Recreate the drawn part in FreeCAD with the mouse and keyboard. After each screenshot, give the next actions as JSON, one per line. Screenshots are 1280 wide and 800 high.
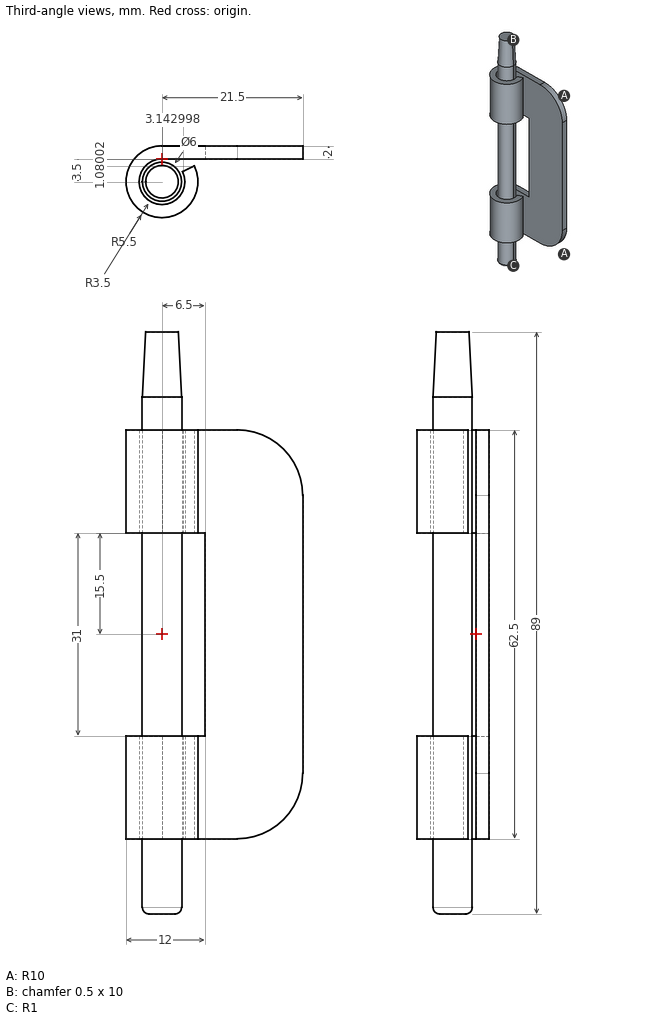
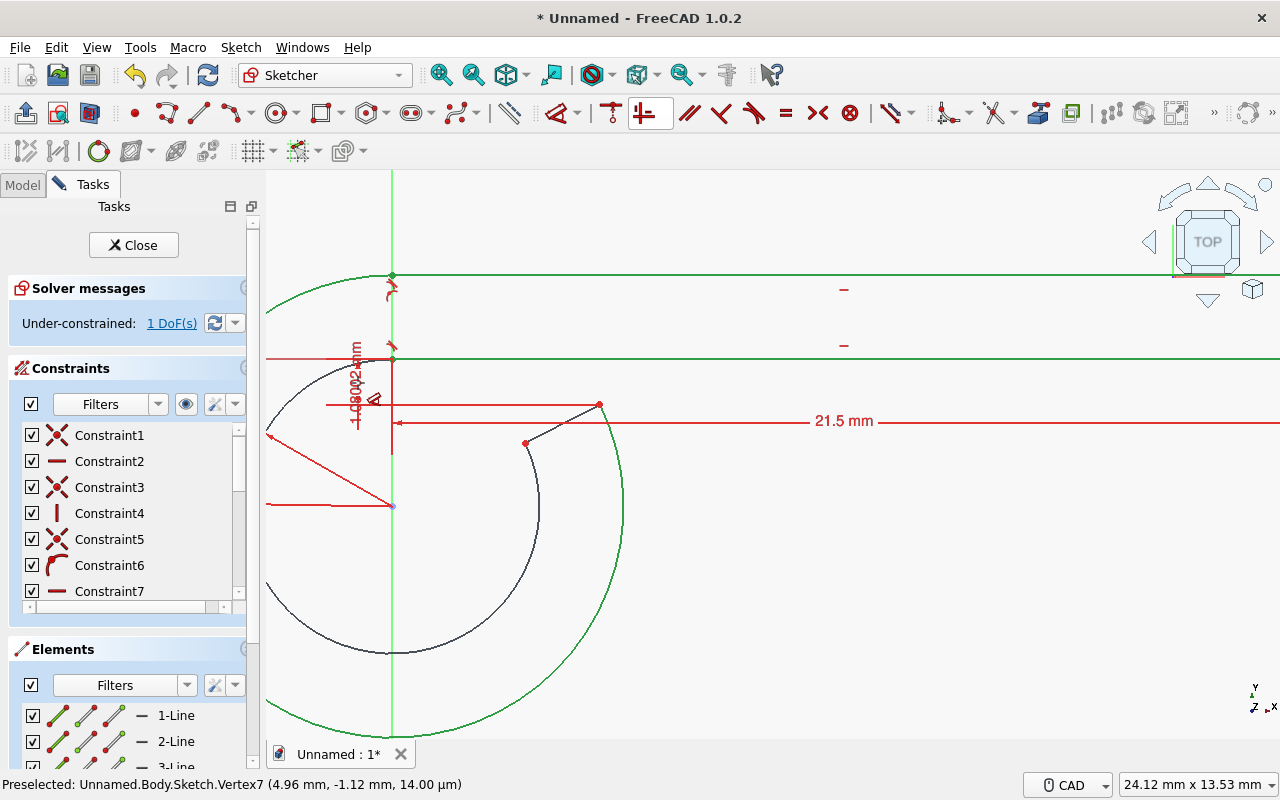
{"action": "left_click", "coordinate": [525, 443]}
{"action": "left_click", "coordinate": [459, 325]}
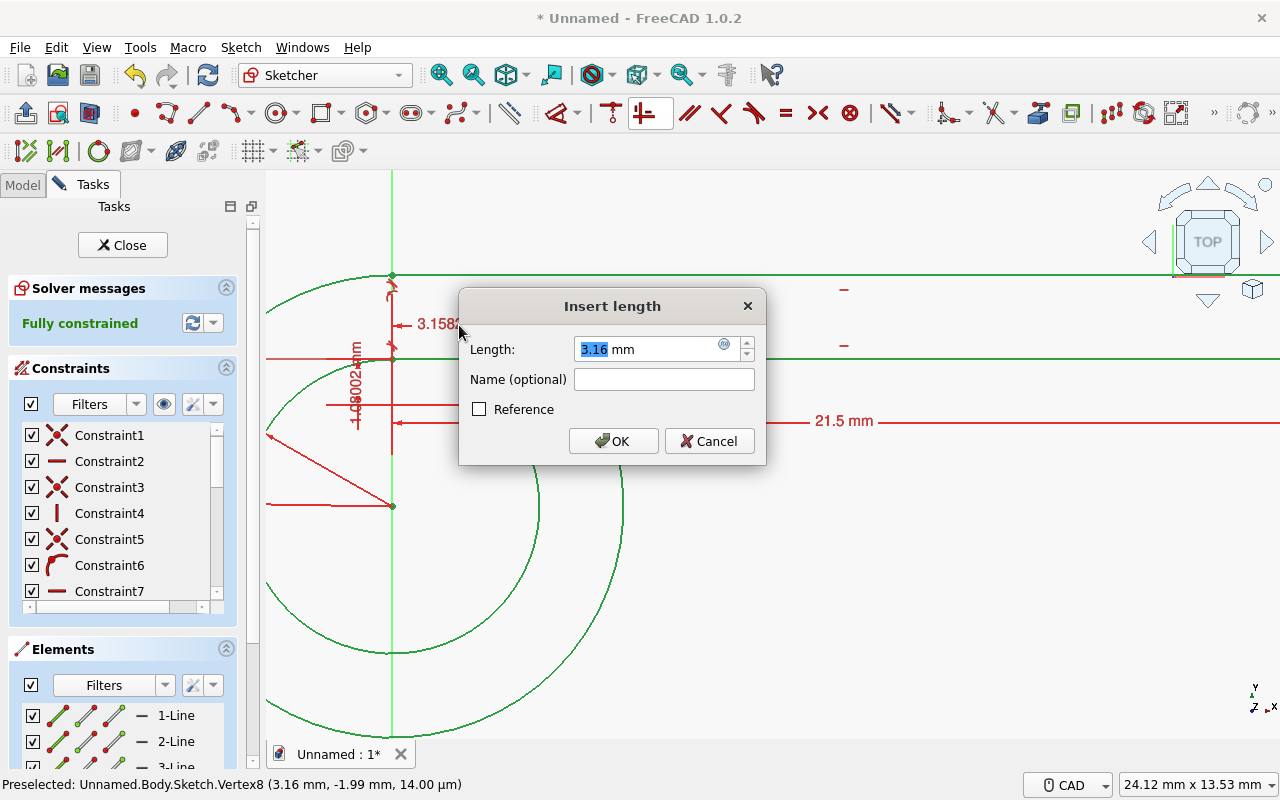
{"action": "type", "text": "3.142998"}
{"action": "key", "text": "Return"}
{"action": "key", "text": "Escape"}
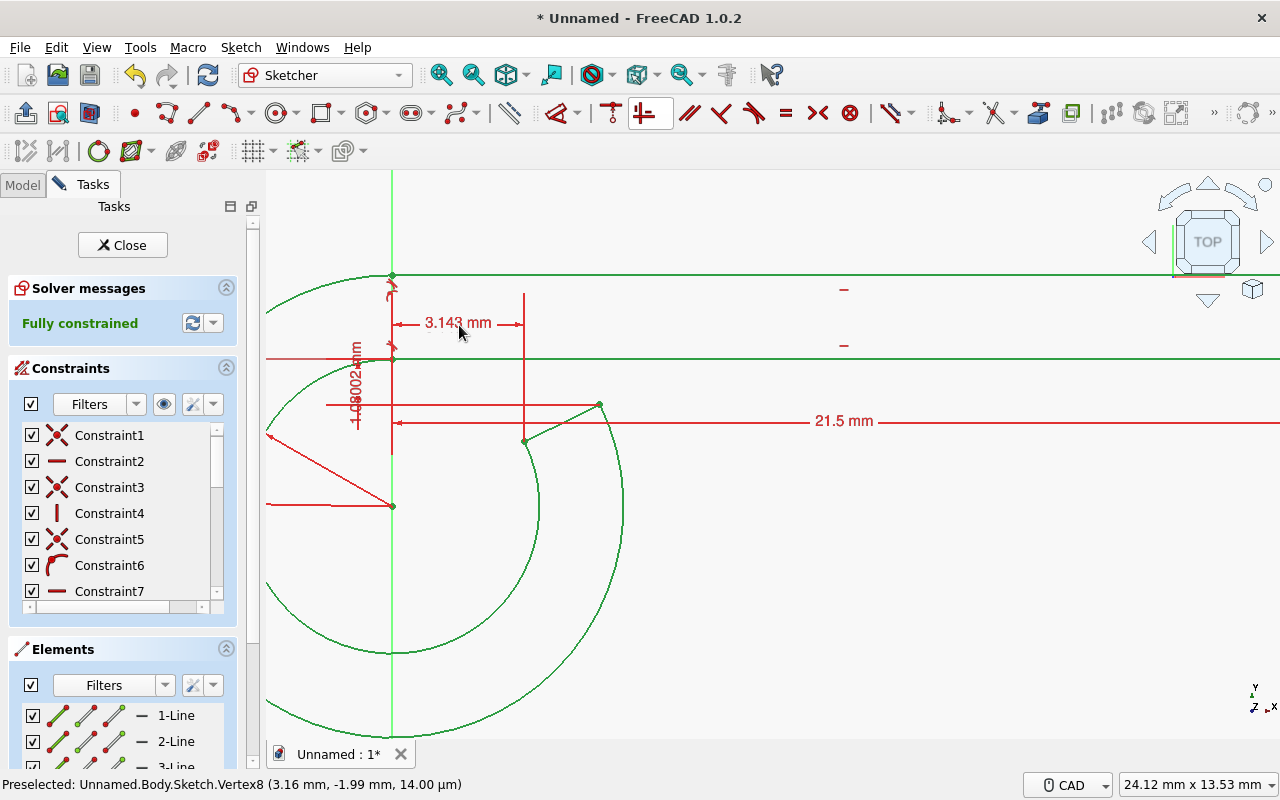
{"action": "left_click", "coordinate": [123, 245]}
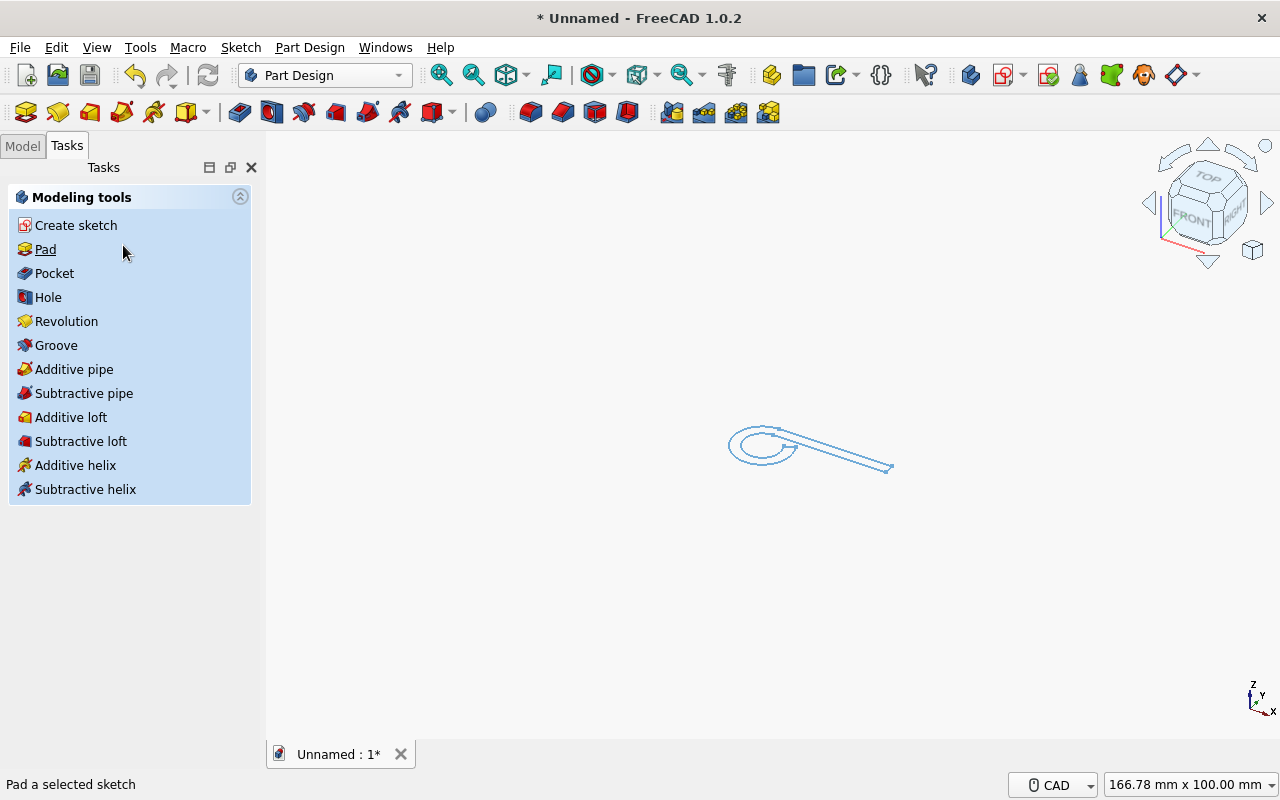
{"action": "left_click", "coordinate": [26, 112]}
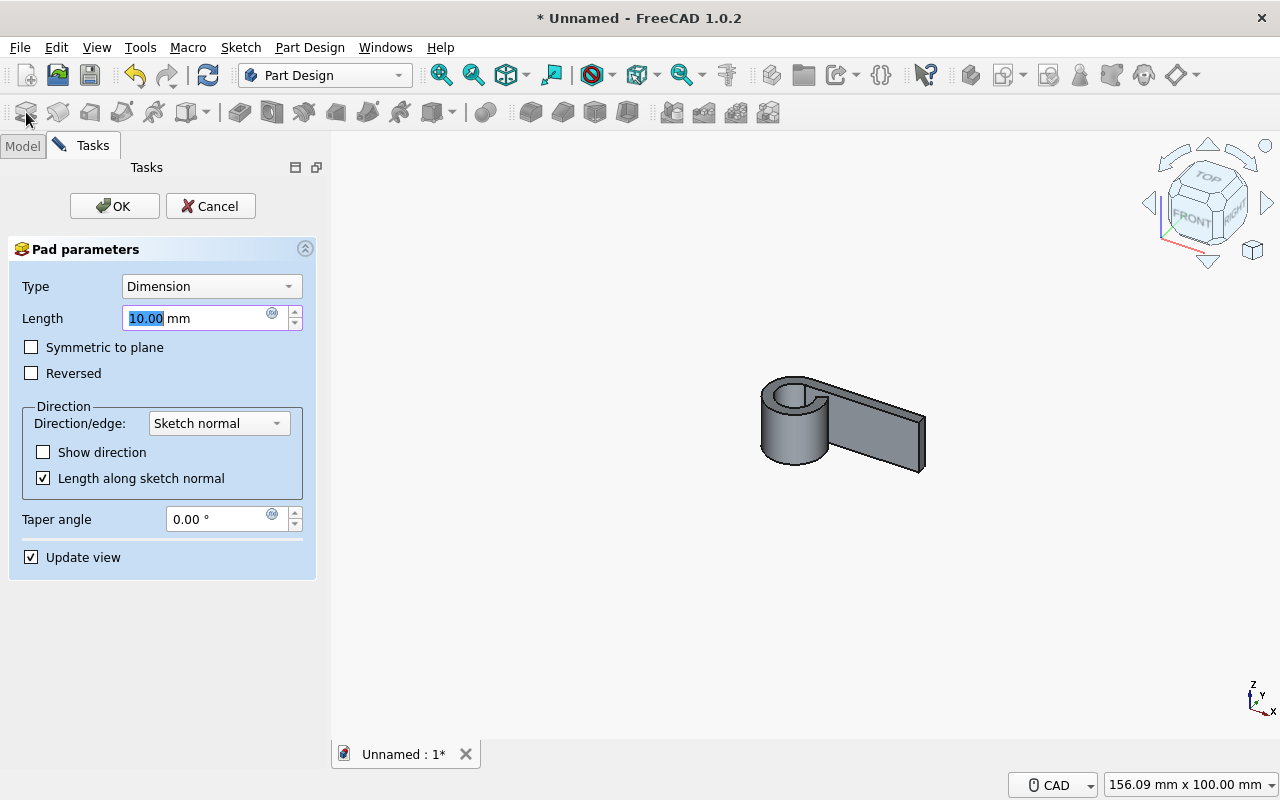
{"action": "type", "text": "62.5"}
{"action": "key", "text": "Tab"}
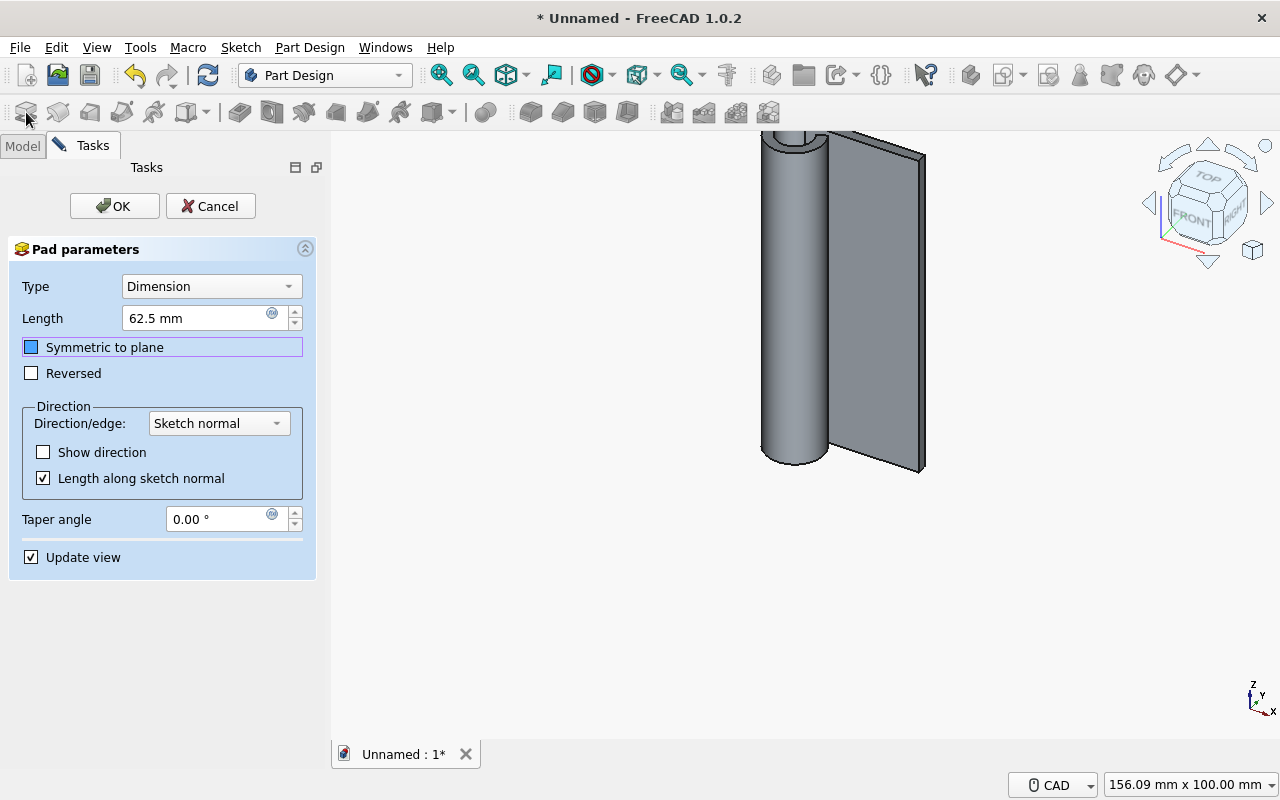
{"action": "left_click", "coordinate": [30, 347]}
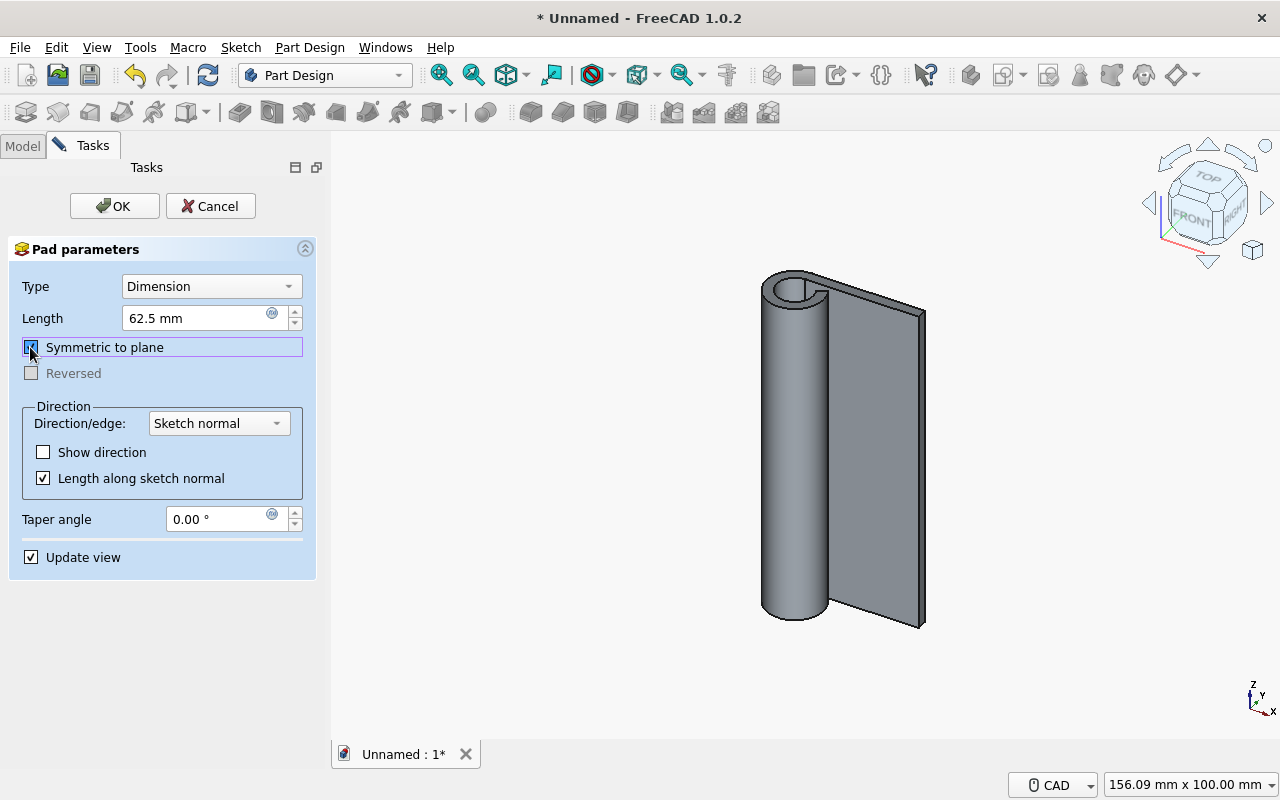
{"action": "left_click", "coordinate": [115, 206]}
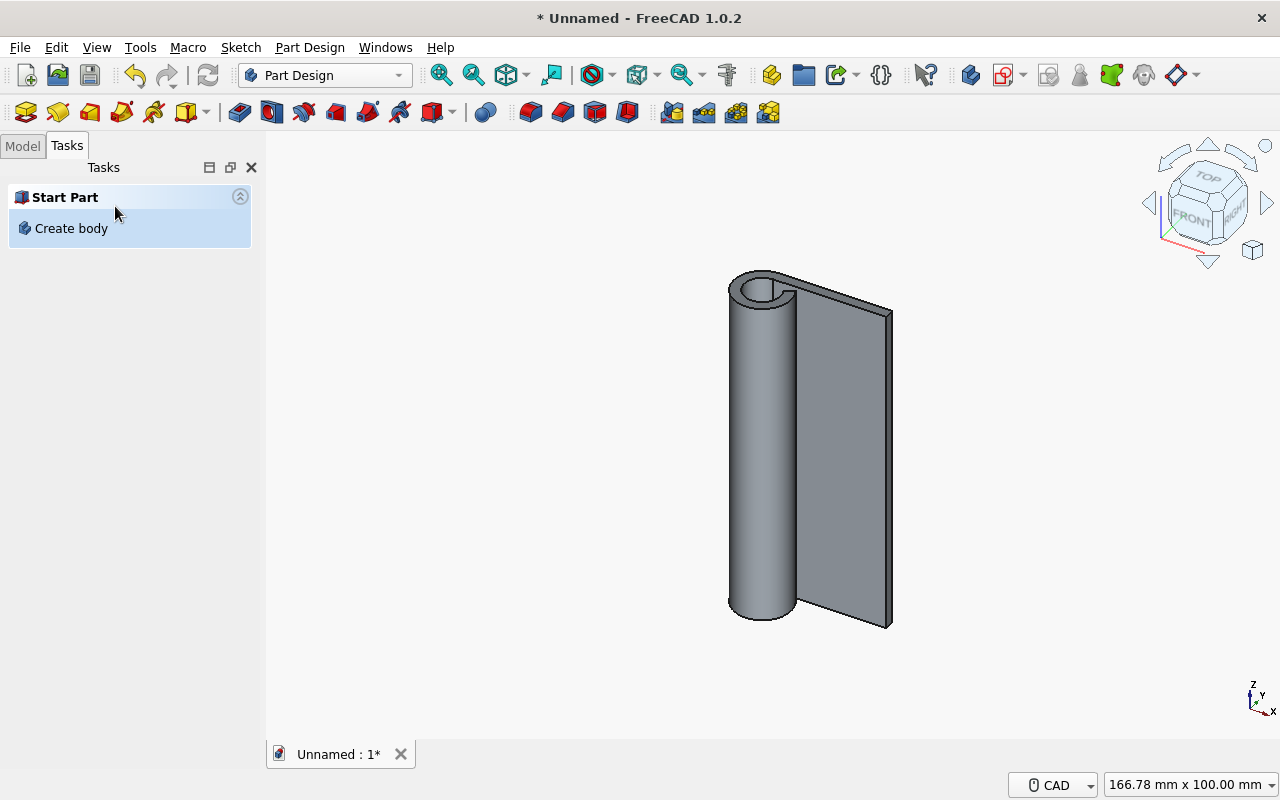
{"action": "key", "text": "4"}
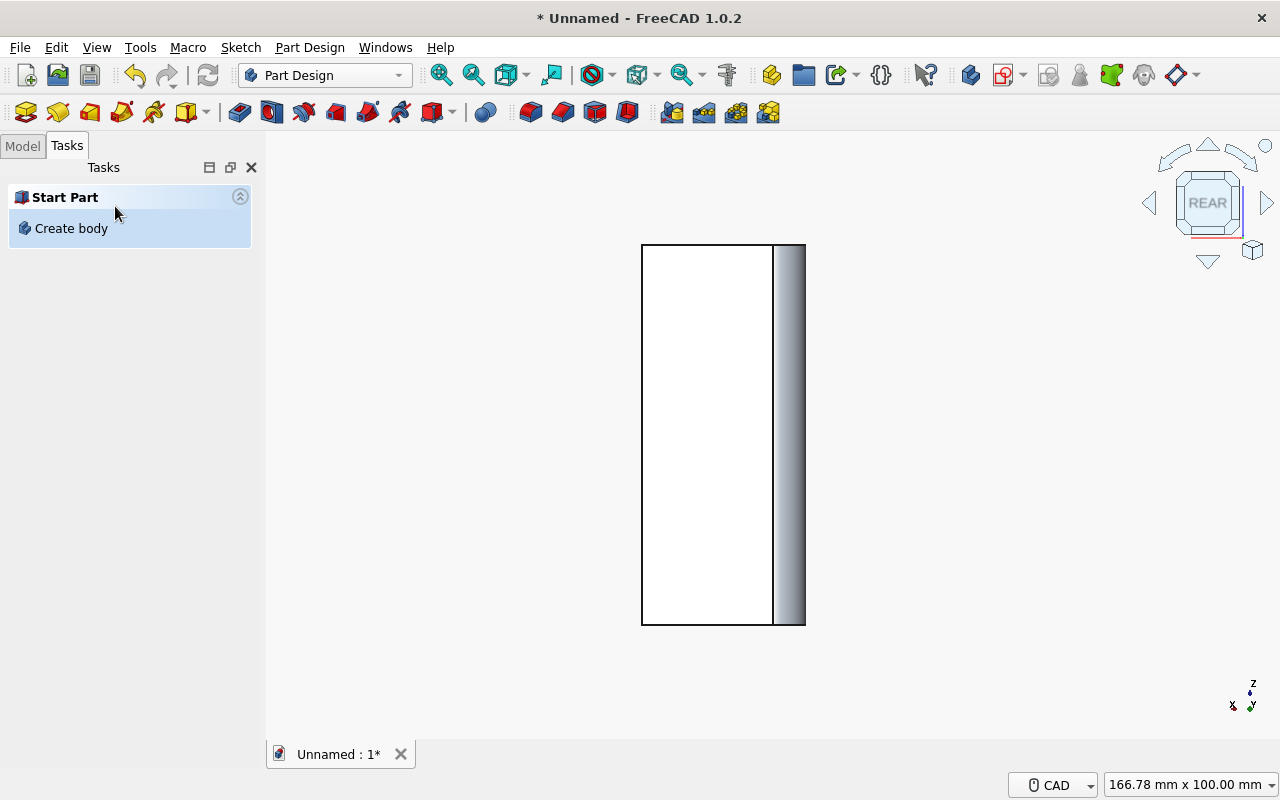
{"action": "left_click", "coordinate": [708, 325]}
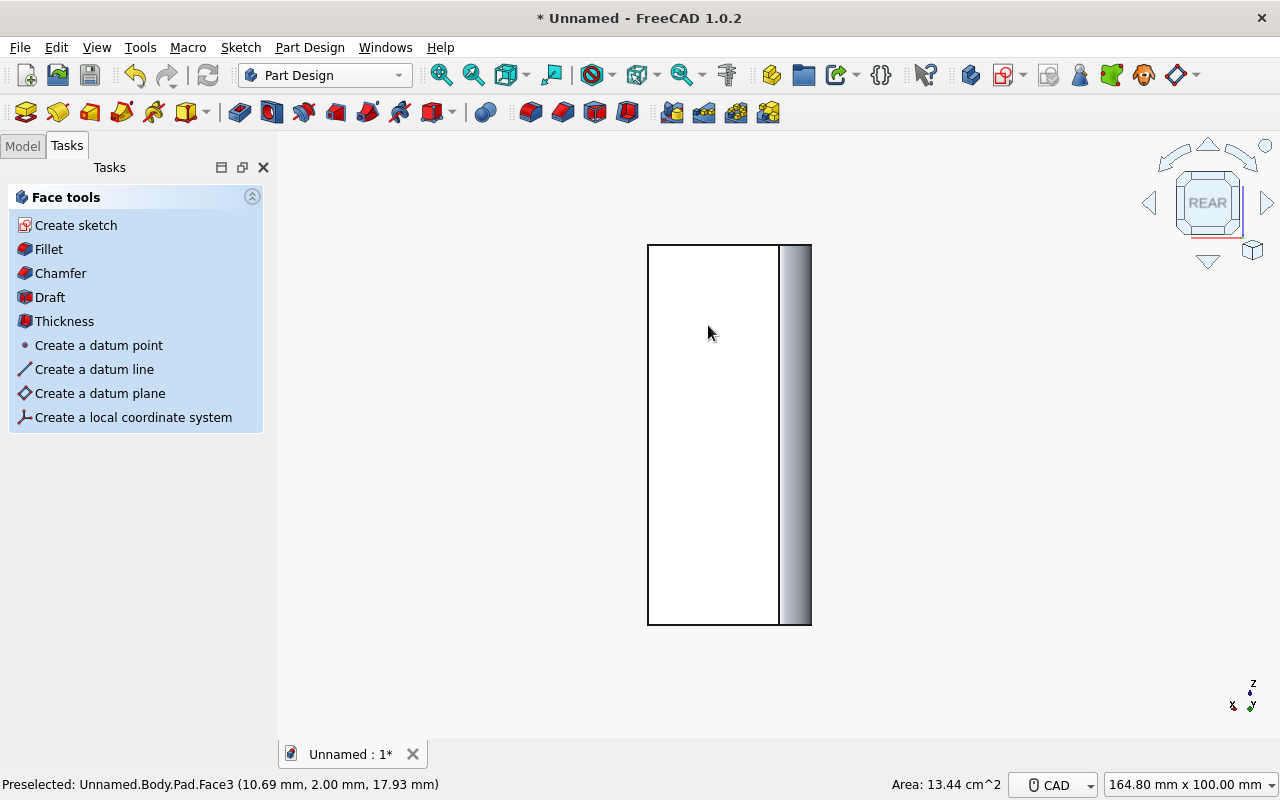
{"action": "left_click", "coordinate": [1004, 76]}